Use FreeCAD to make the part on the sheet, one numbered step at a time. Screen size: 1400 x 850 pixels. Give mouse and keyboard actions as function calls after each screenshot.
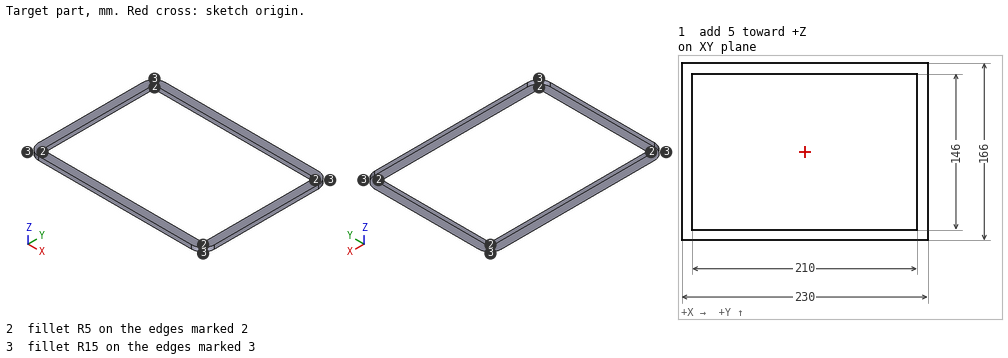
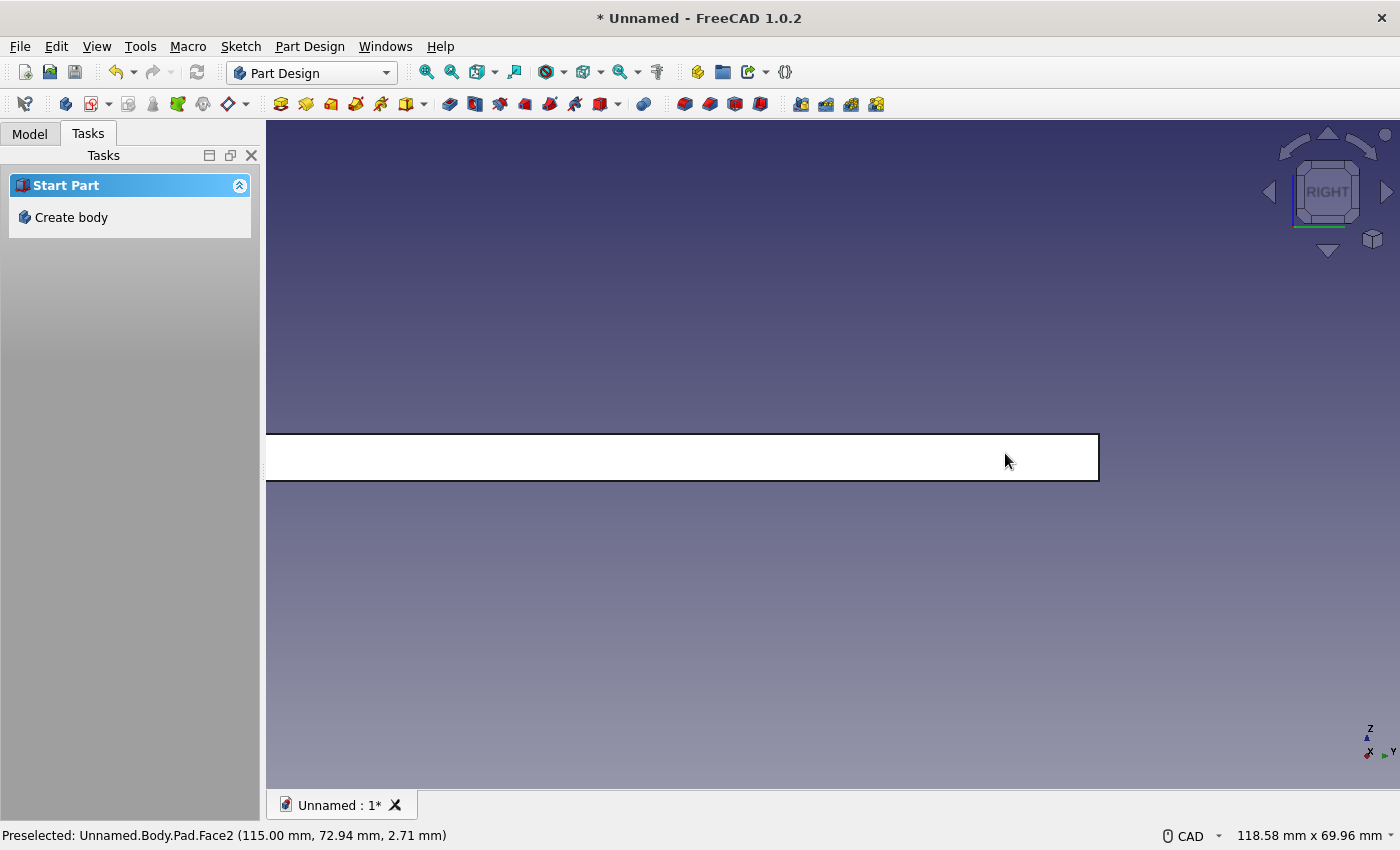
key(v)
key(f)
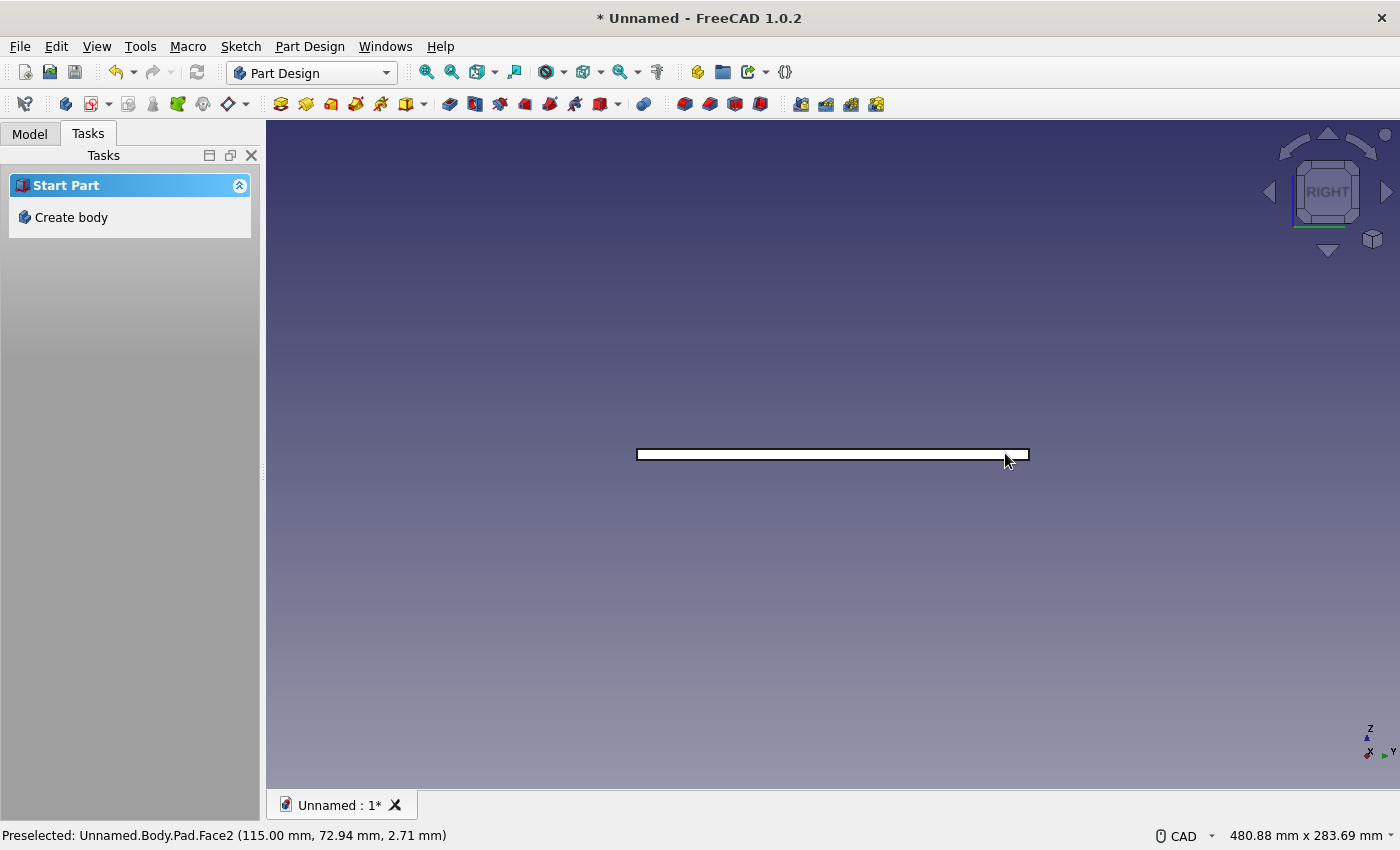
key(5)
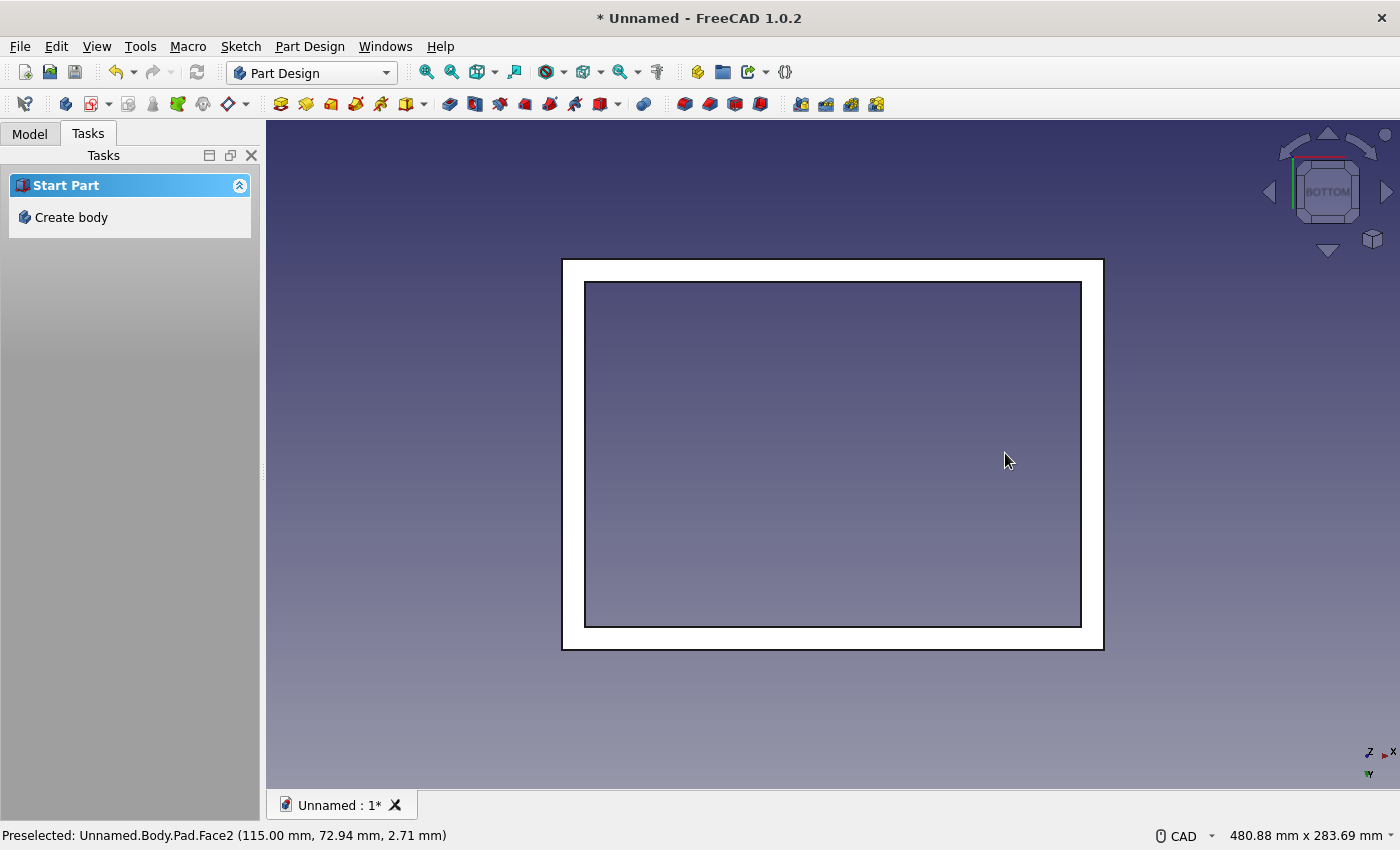
scroll(585, 626, up, 7)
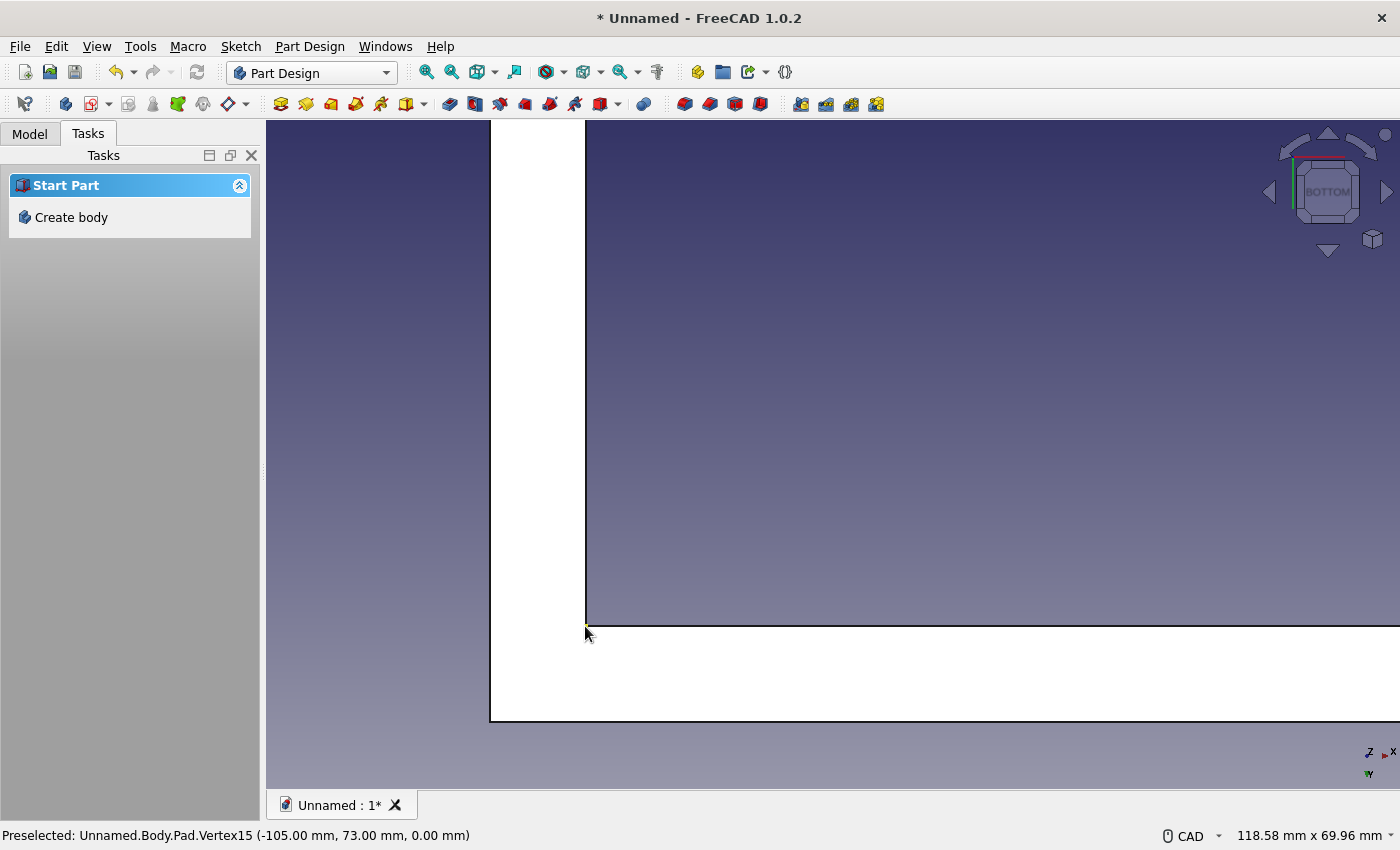
key(v)
key(f)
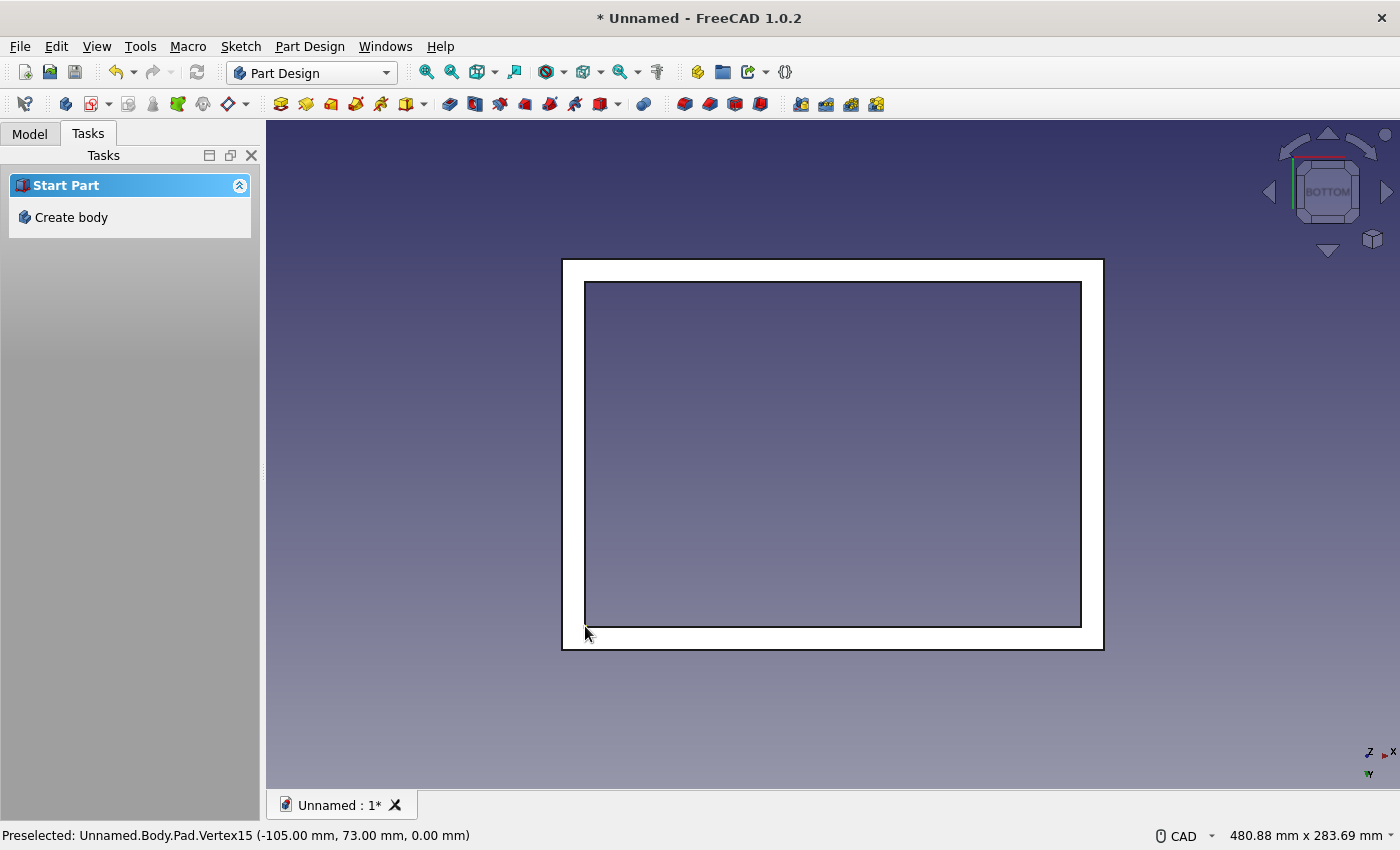
key(4)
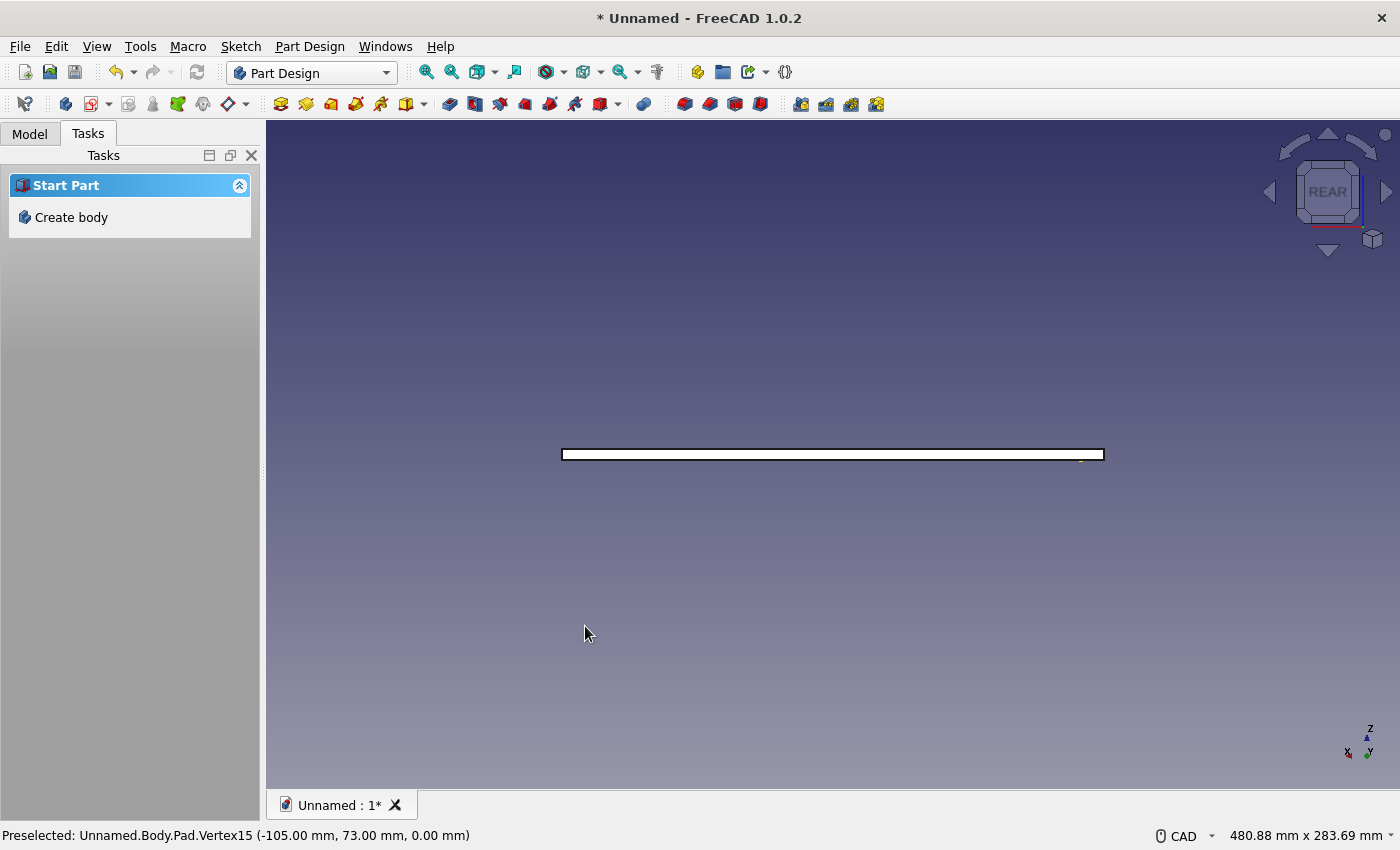
scroll(1081, 453, up, 7)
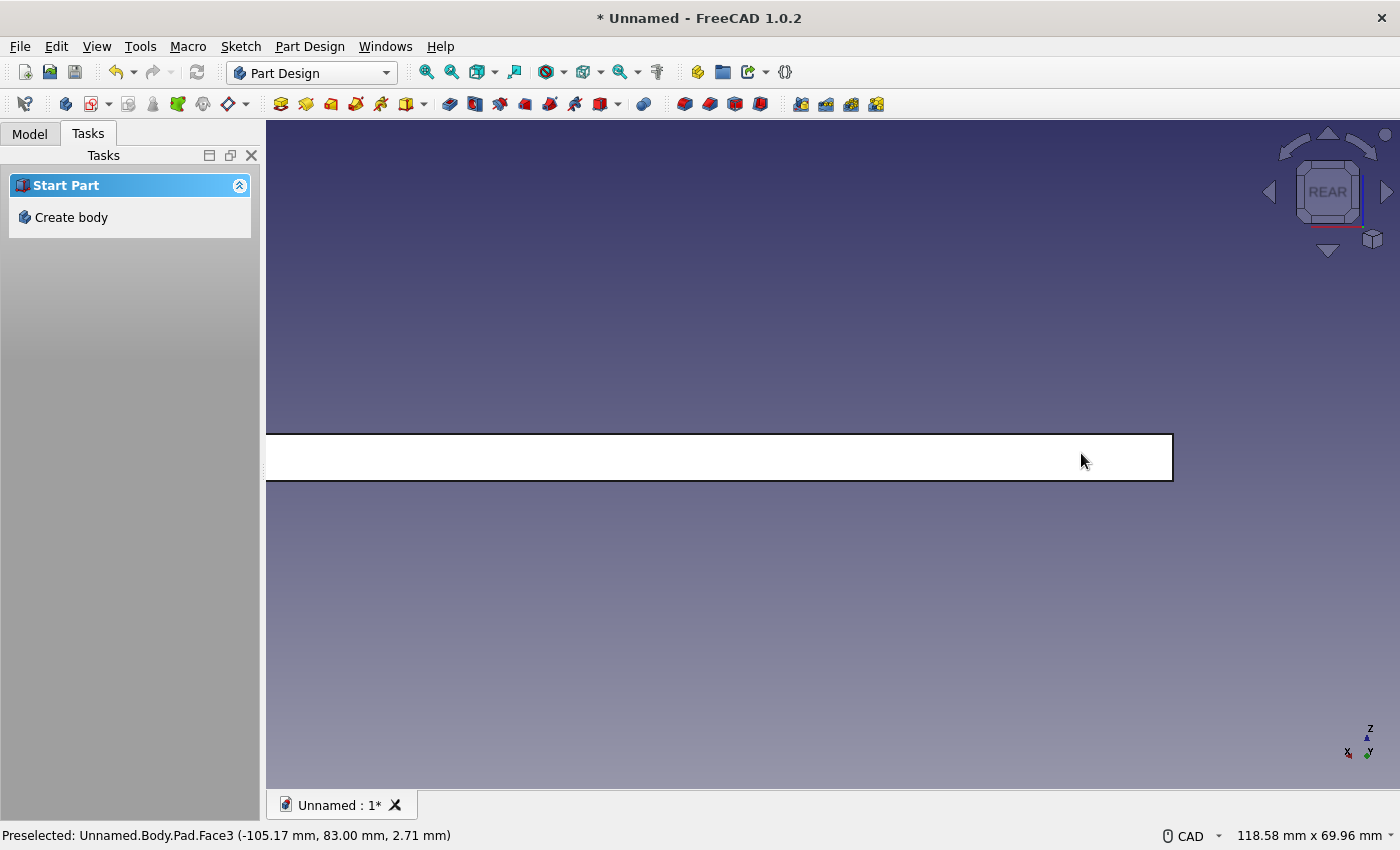
click(427, 72)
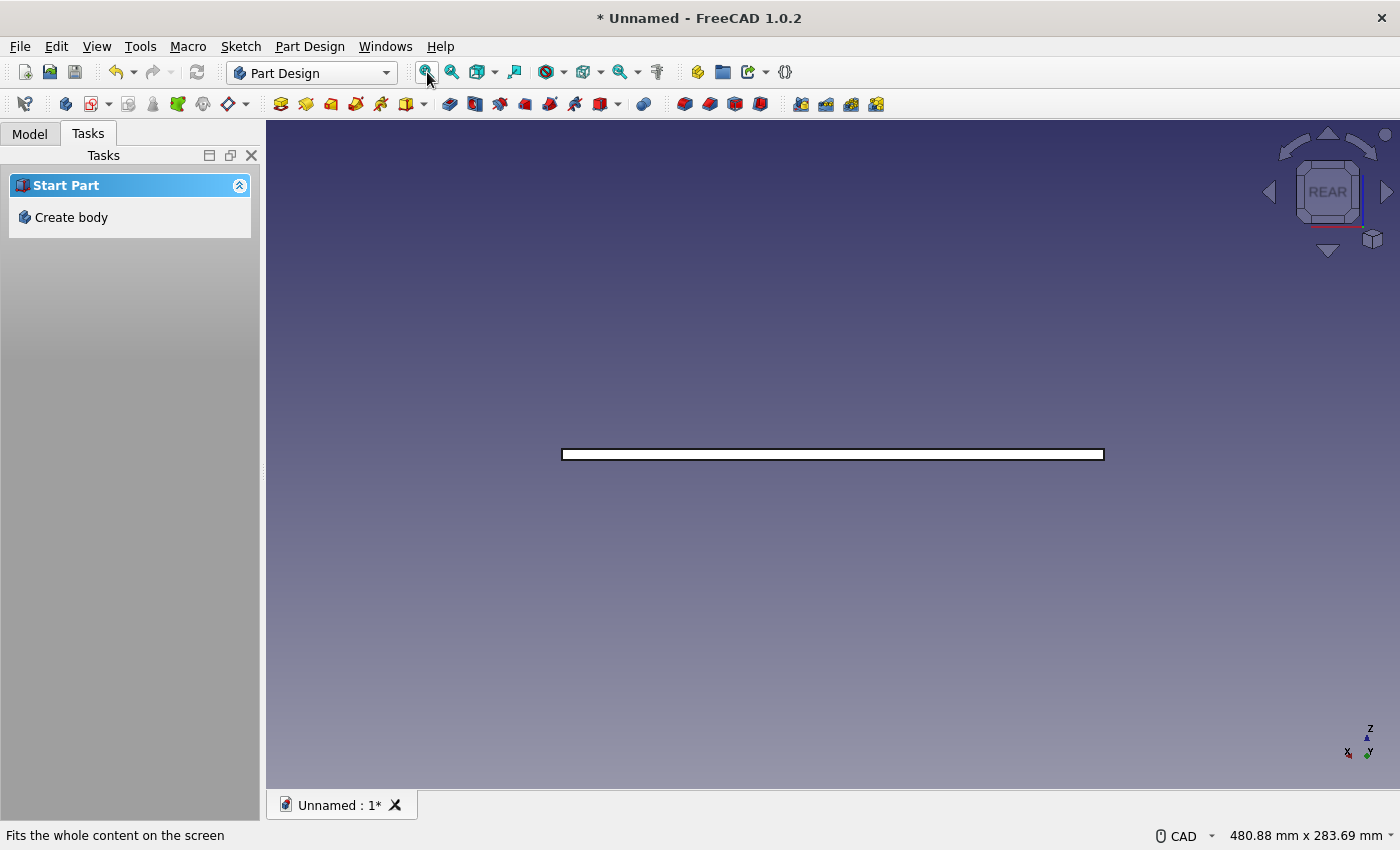
key(6)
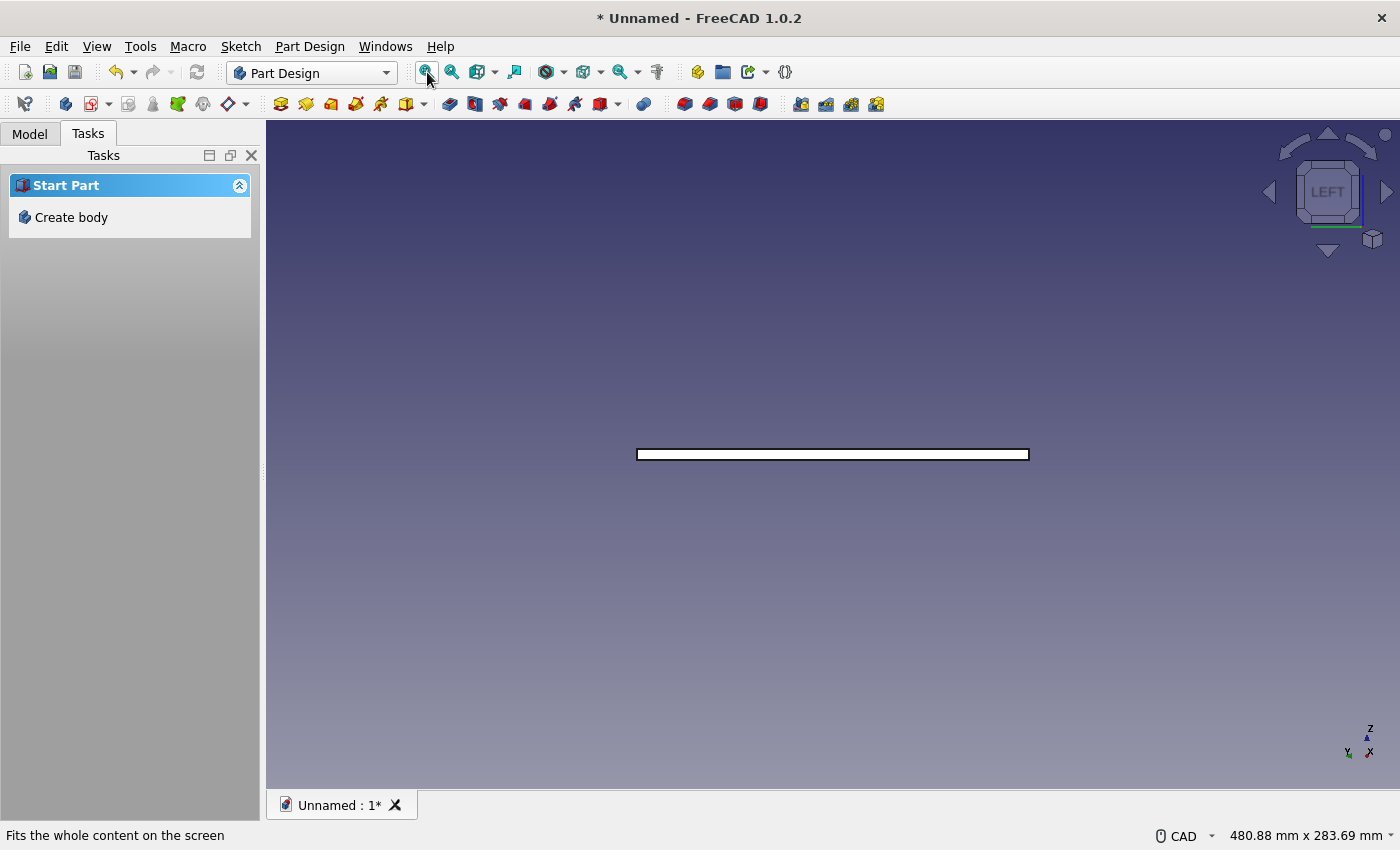
click(427, 72)